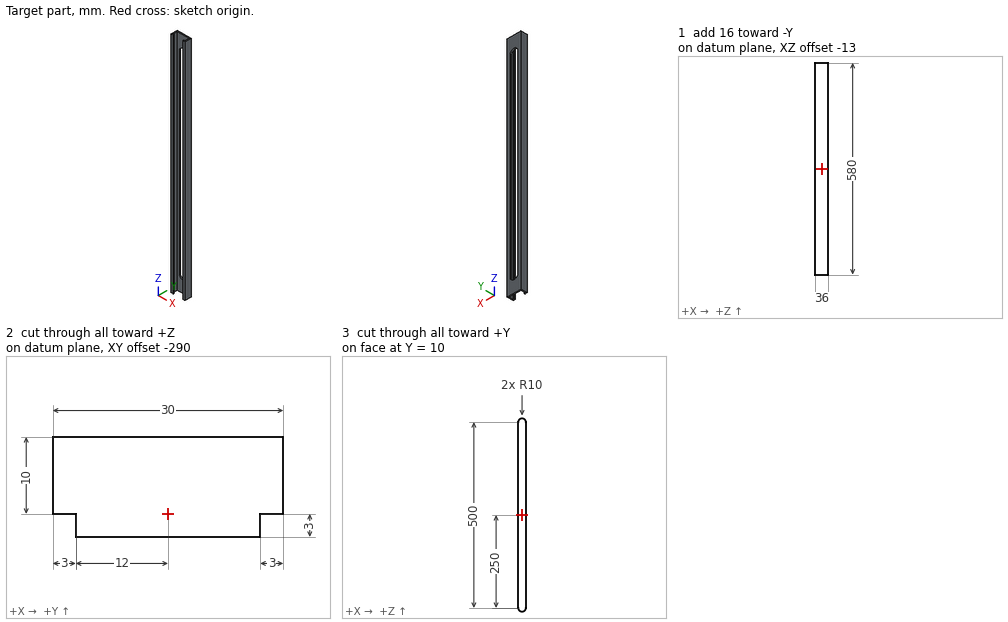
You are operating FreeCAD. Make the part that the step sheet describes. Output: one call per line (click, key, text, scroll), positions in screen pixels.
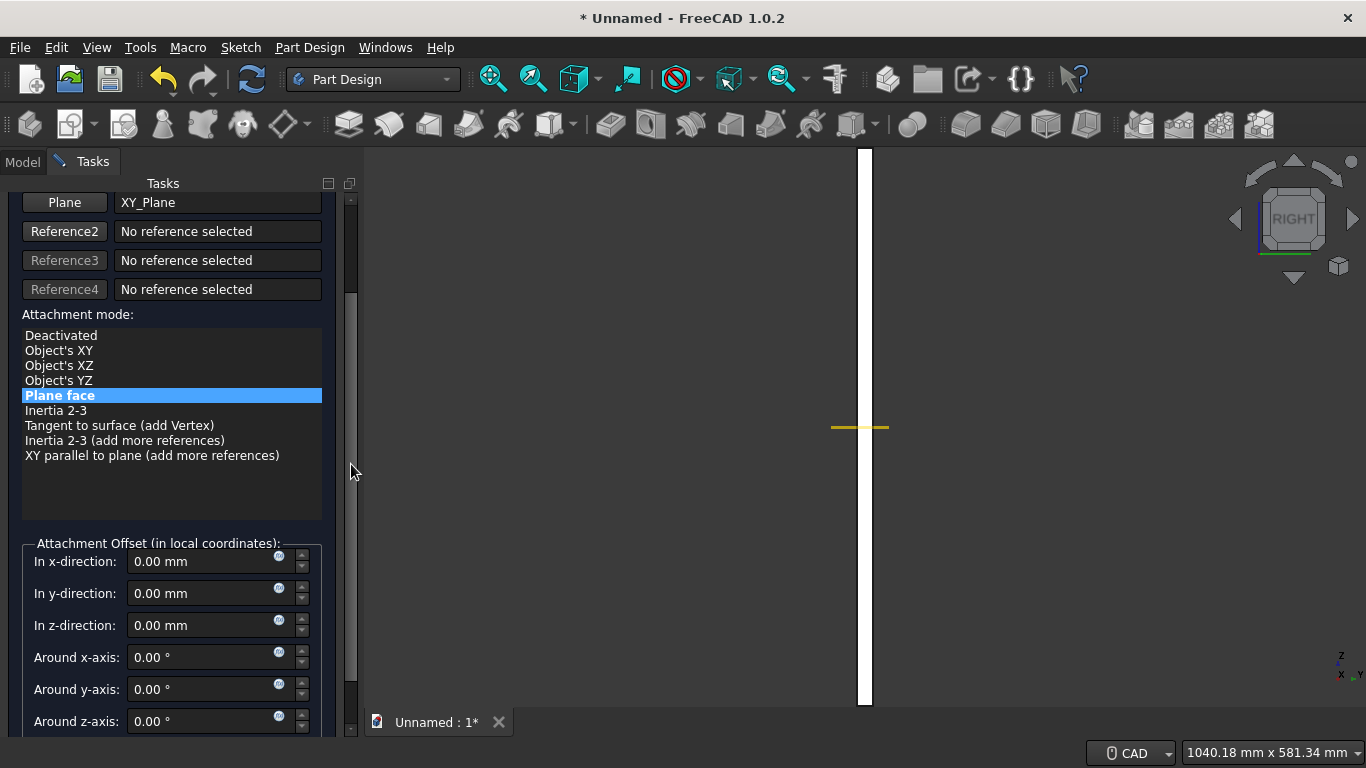
triple_click(210, 625)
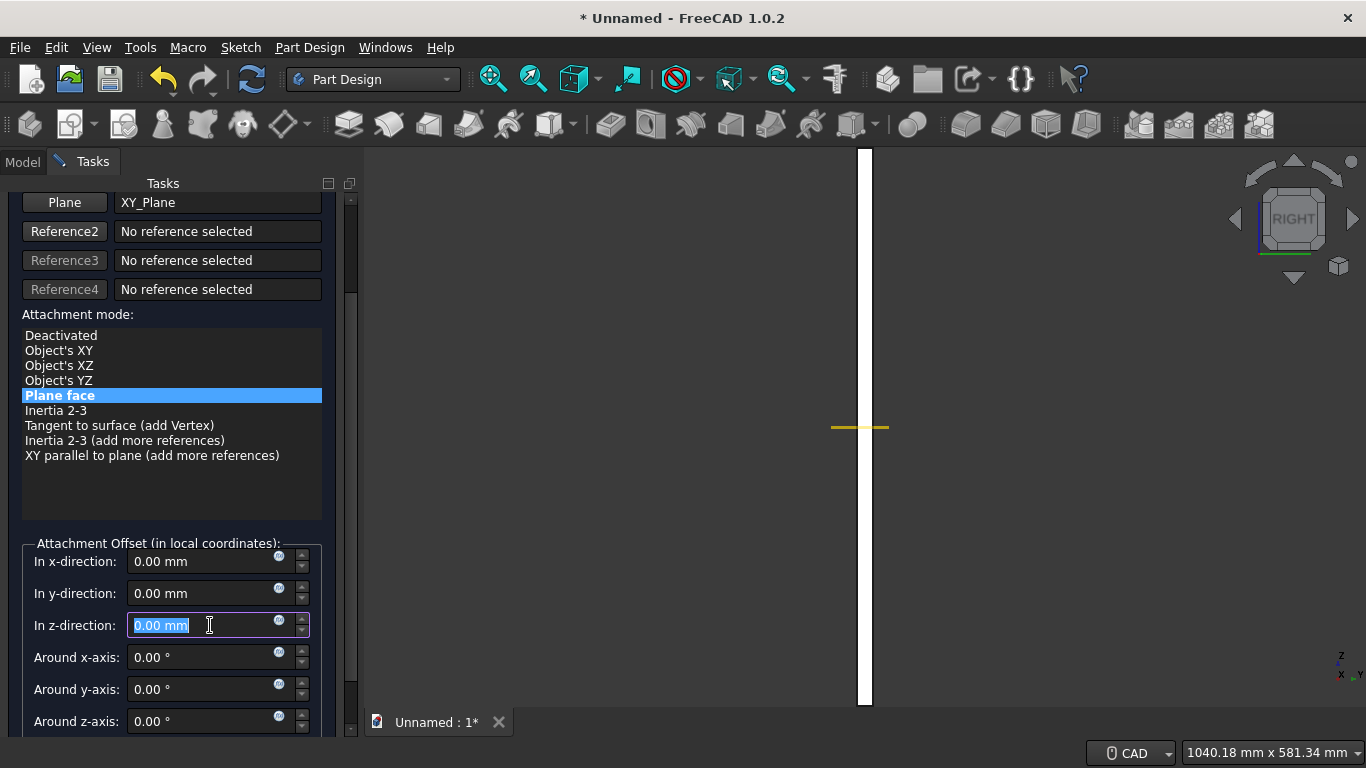
text(-290)
key(Tab)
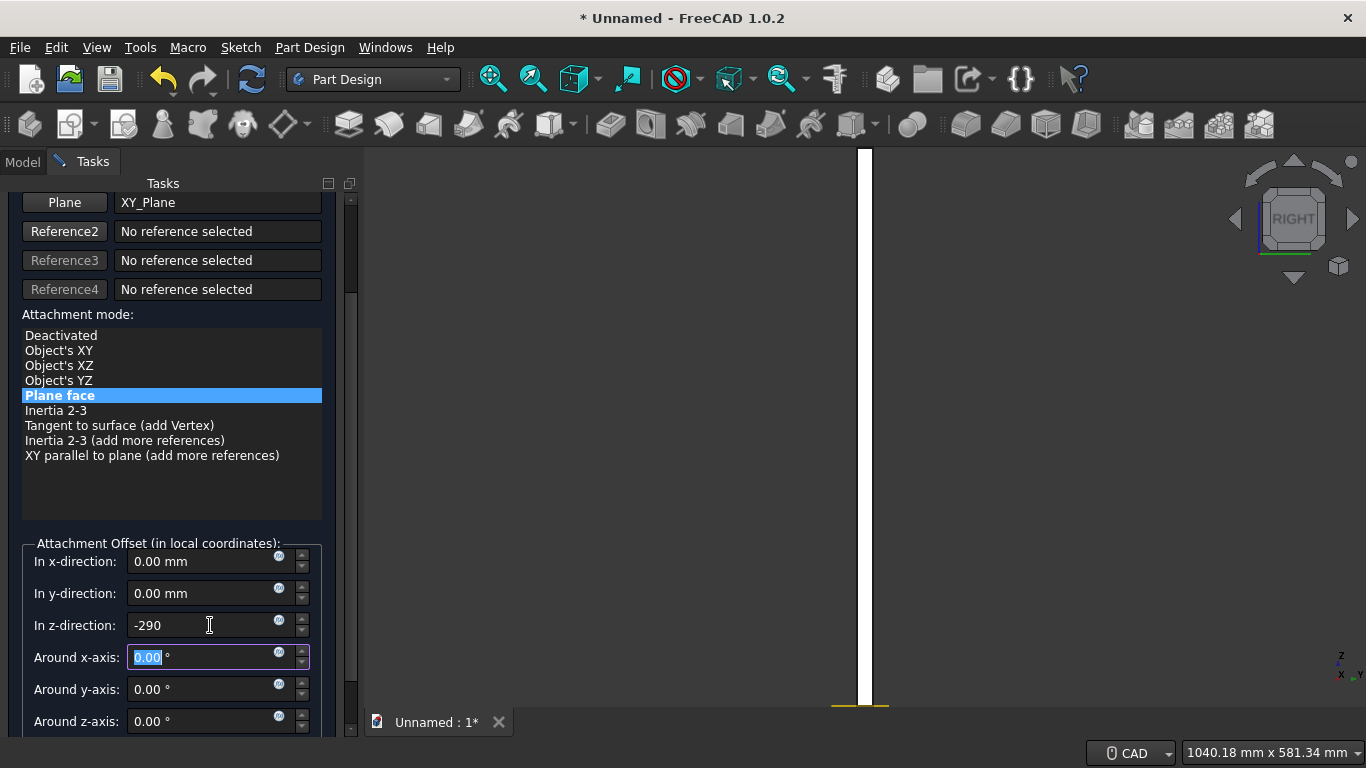
scroll(351, 464, up, 3)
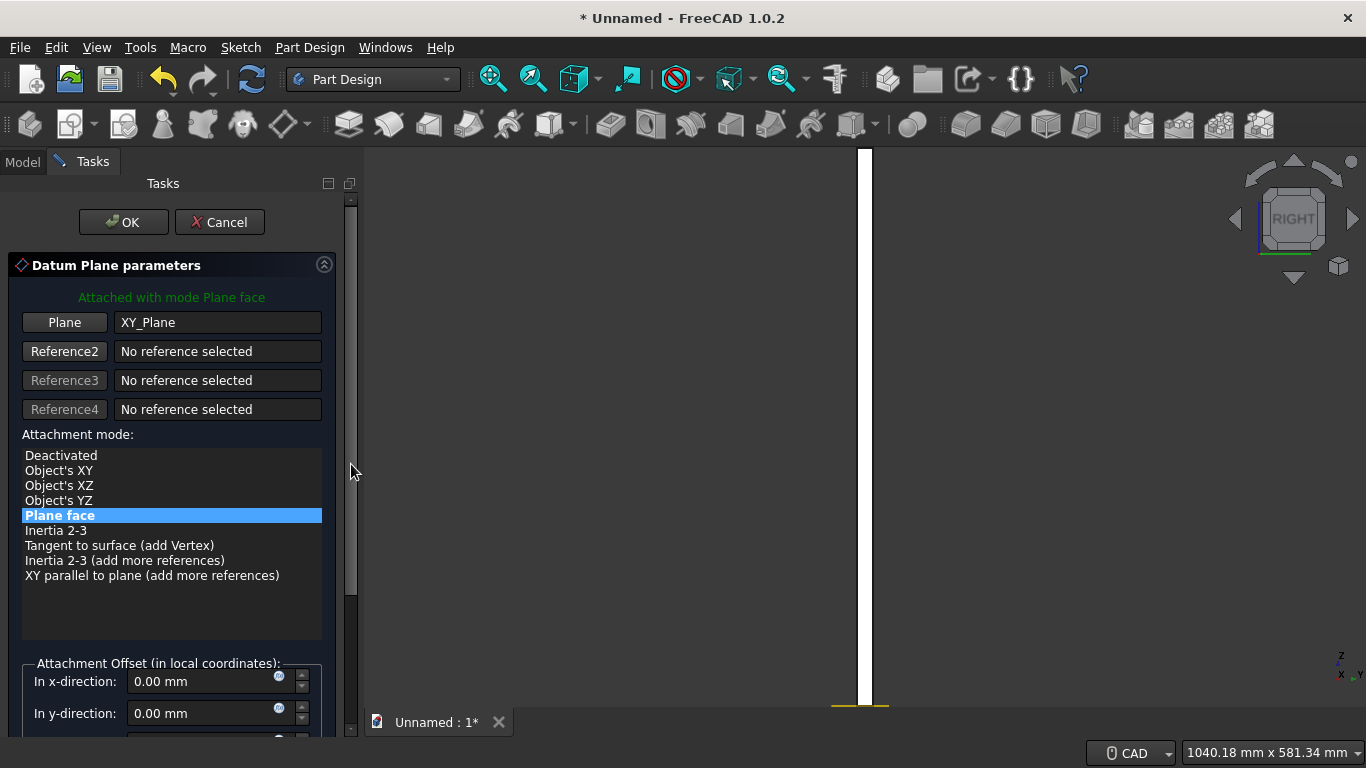
click(124, 222)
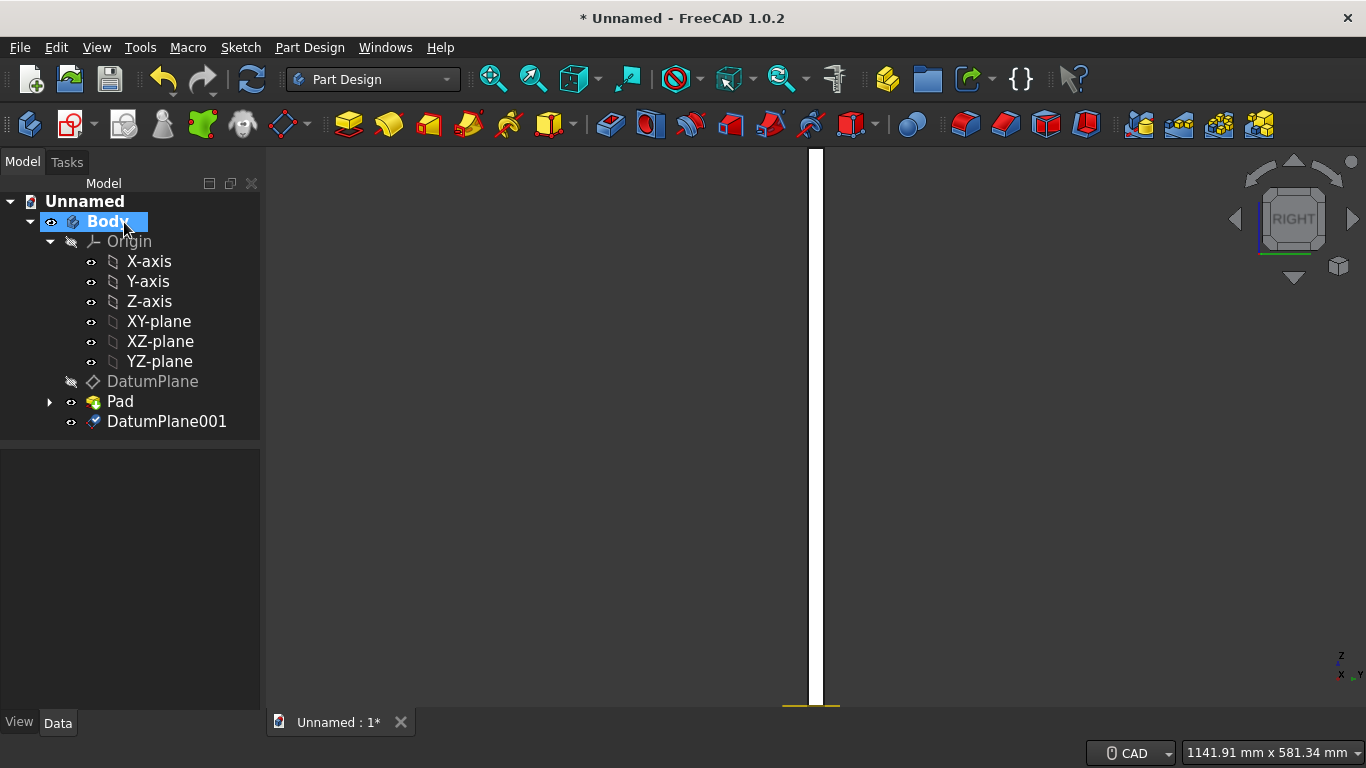
click(116, 422)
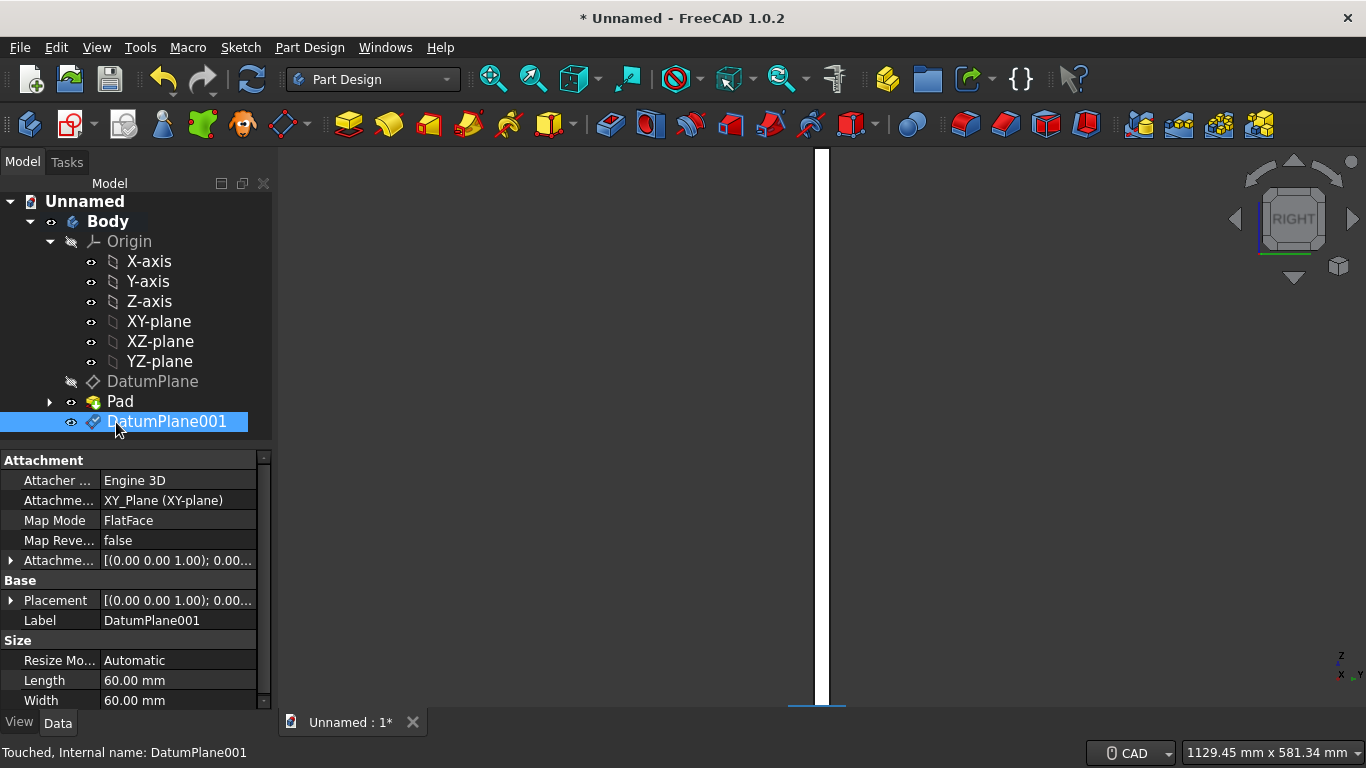
click(70, 124)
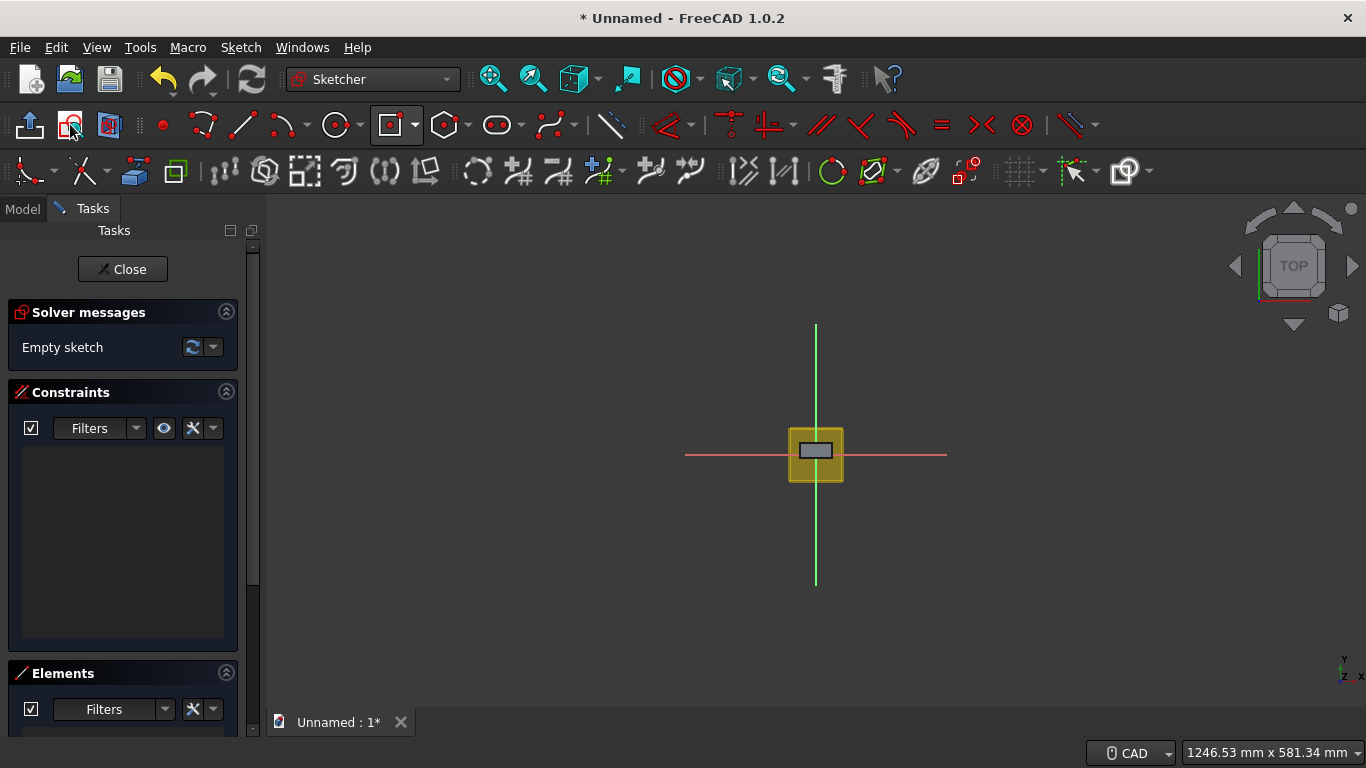
click(110, 126)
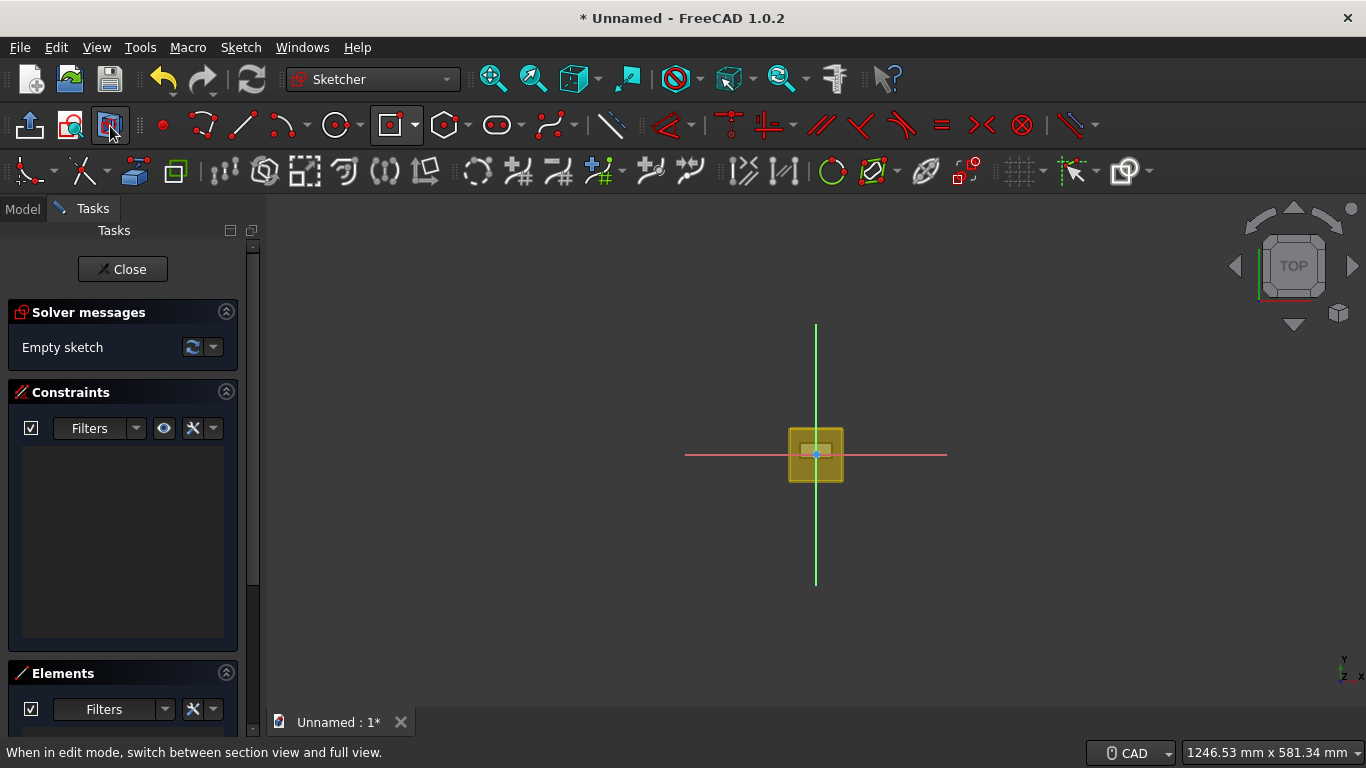
scroll(820, 452, up, 15)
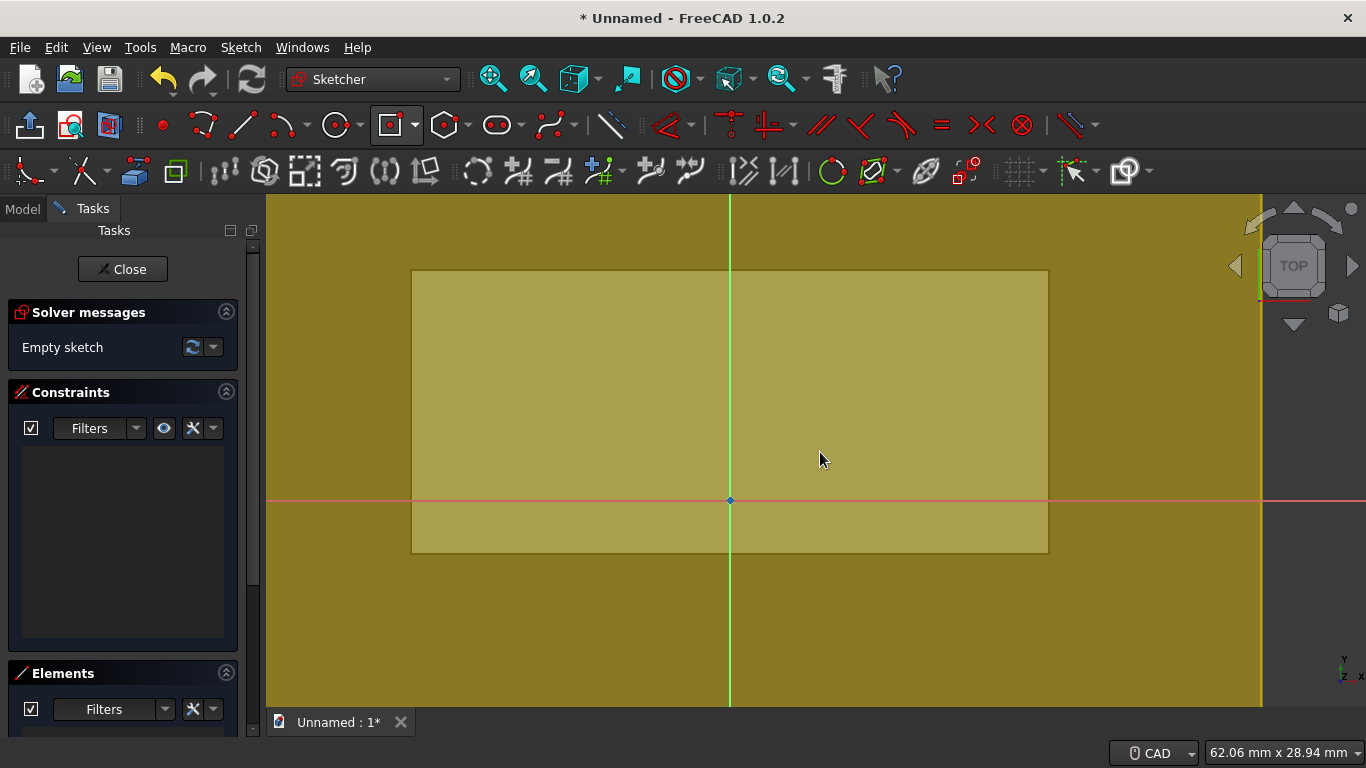
click(204, 126)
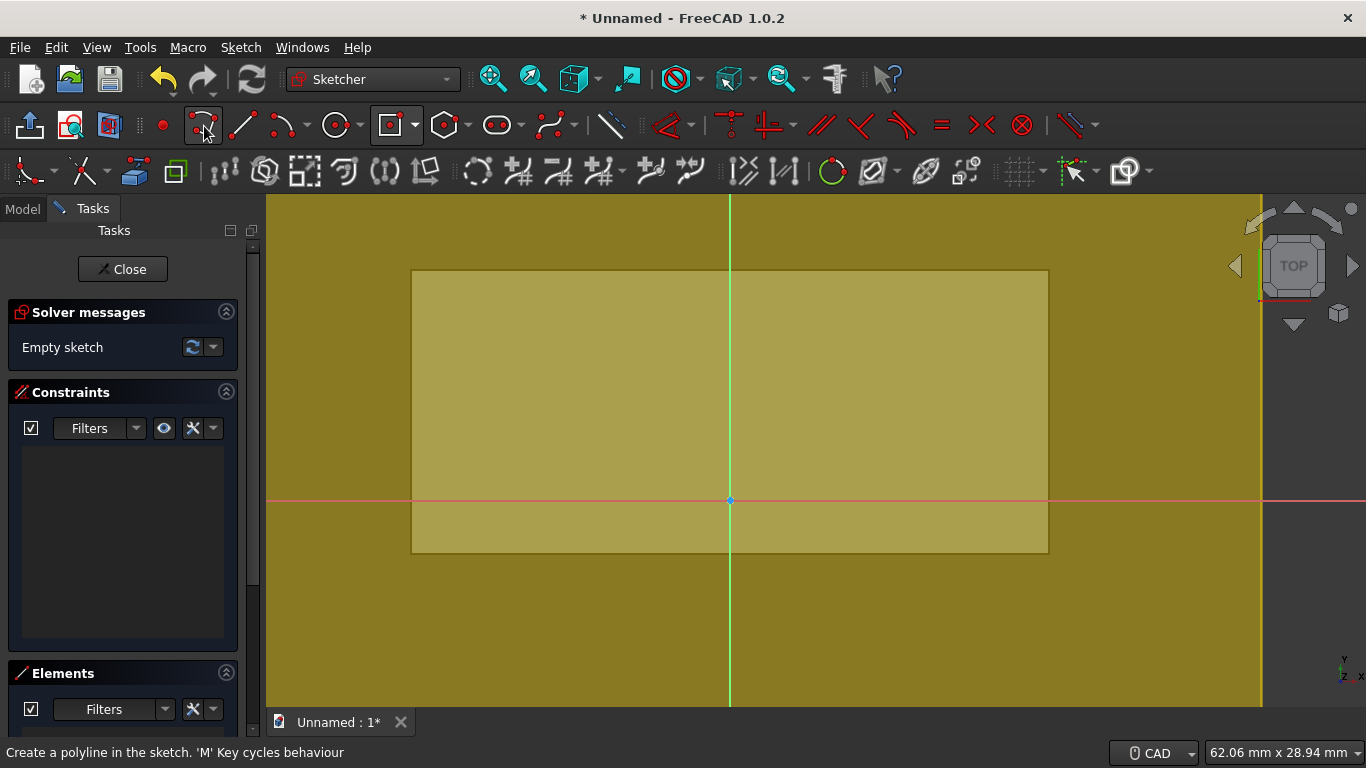
click(517, 501)
click(464, 492)
click(464, 324)
click(996, 324)
click(996, 501)
click(943, 492)
click(943, 554)
click(517, 554)
click(517, 501)
key(Escape)
key(Escape)